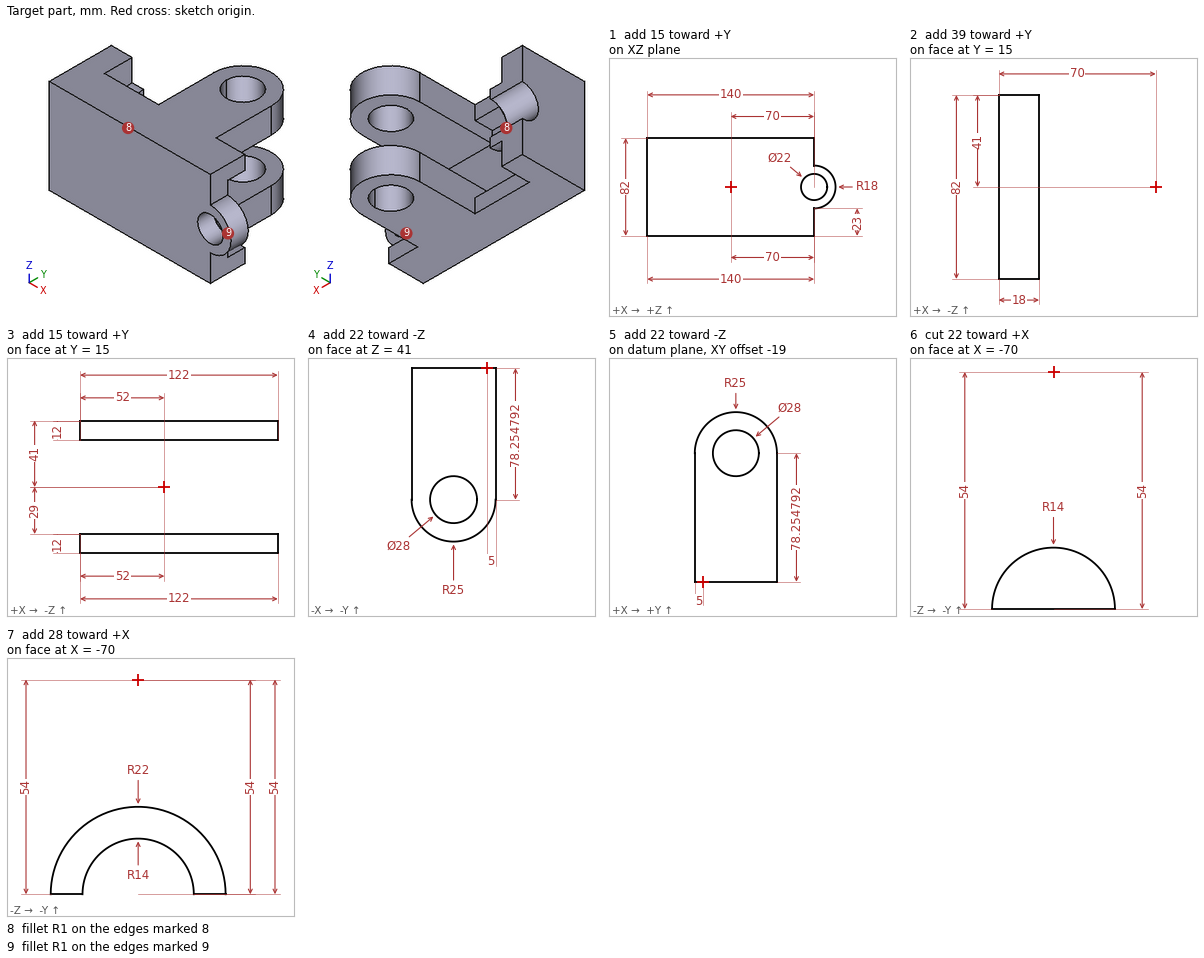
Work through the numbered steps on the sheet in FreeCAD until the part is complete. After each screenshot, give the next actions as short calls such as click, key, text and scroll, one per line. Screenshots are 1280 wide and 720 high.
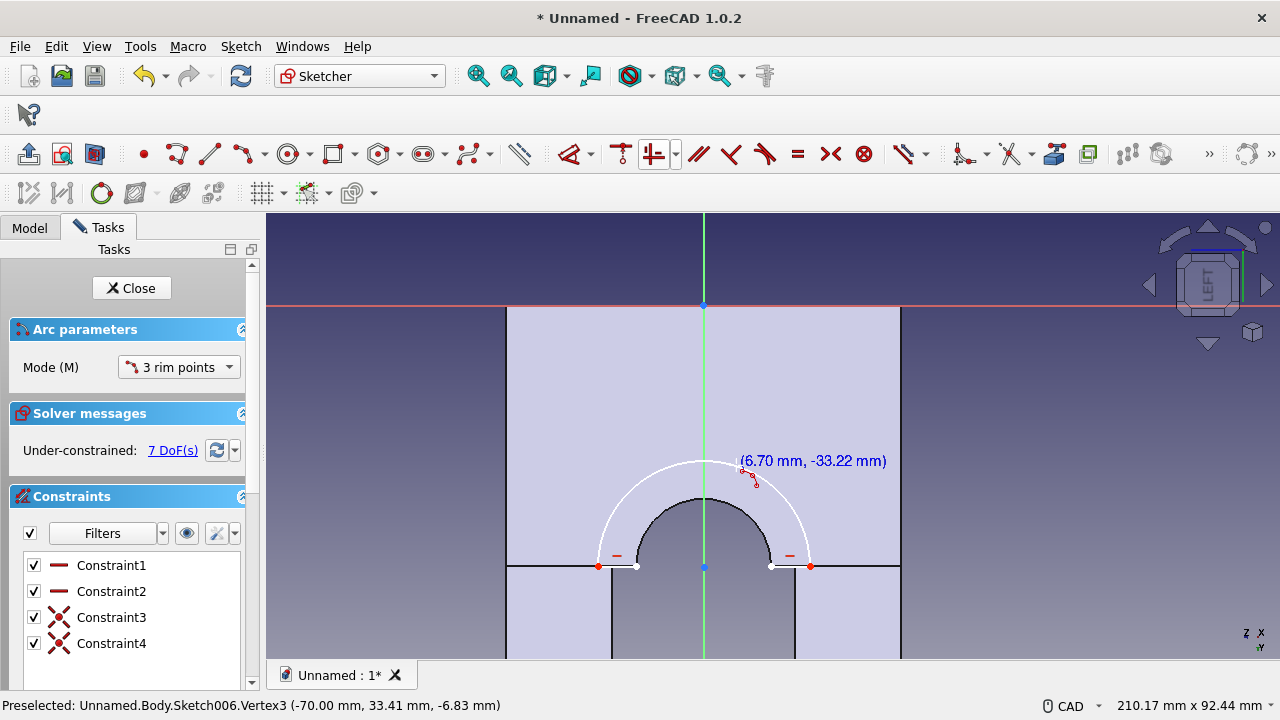
click(636, 567)
click(771, 567)
click(725, 502)
key(Escape)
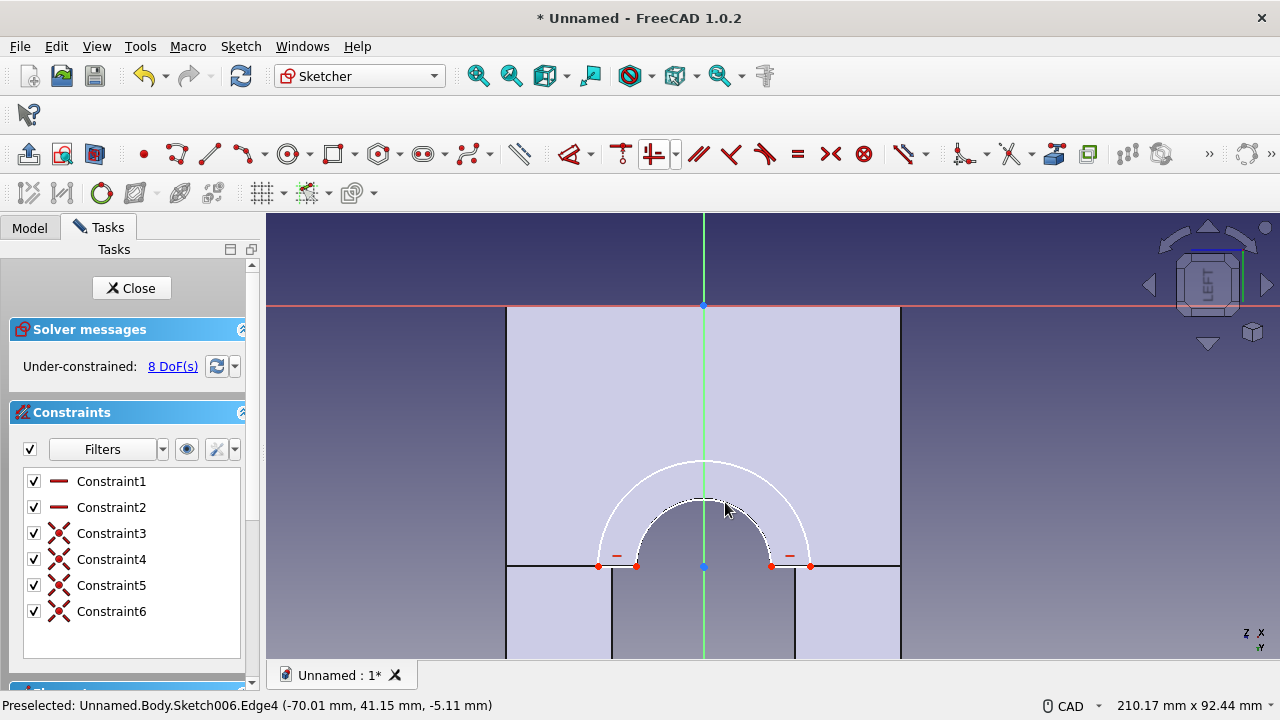
click(766, 481)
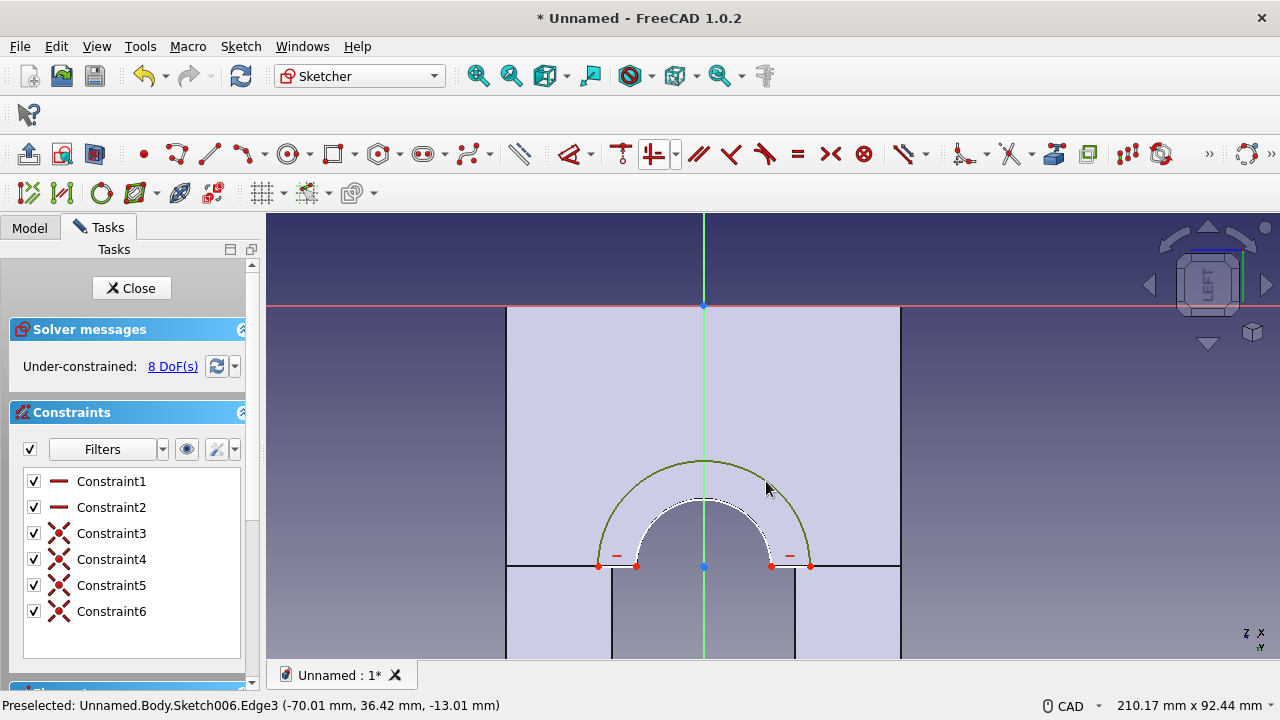
click(743, 512)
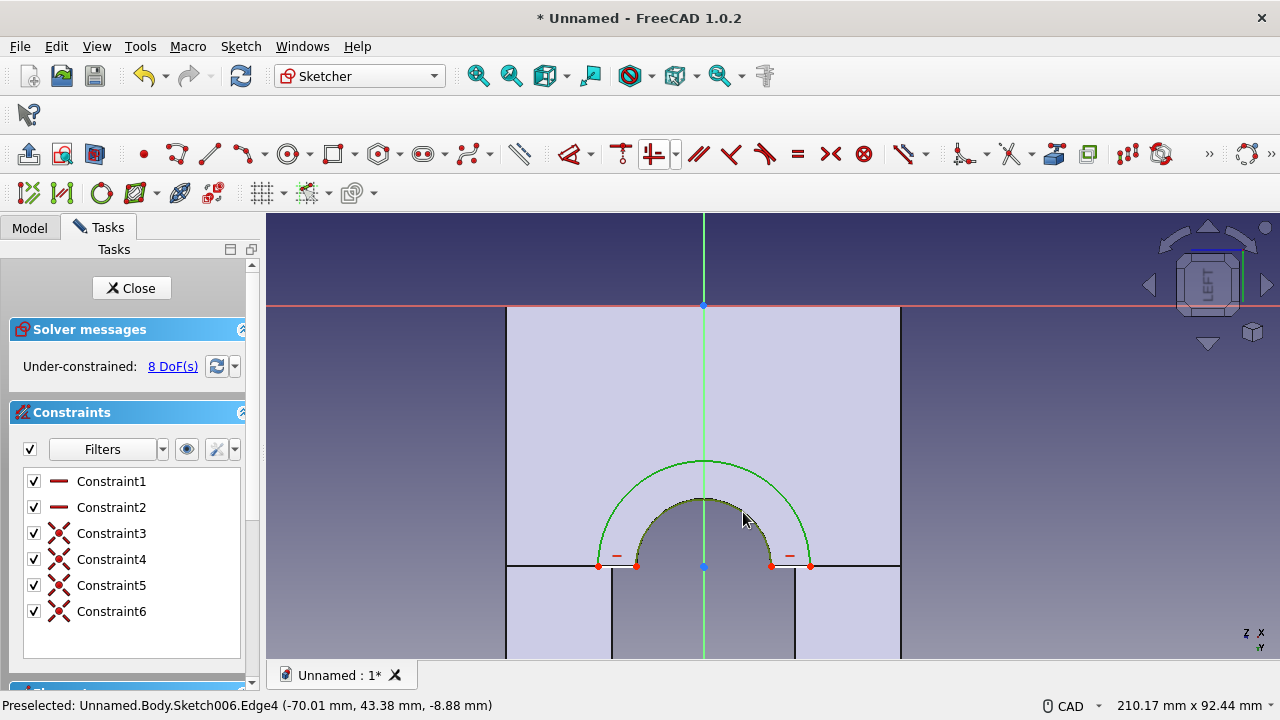
click(621, 154)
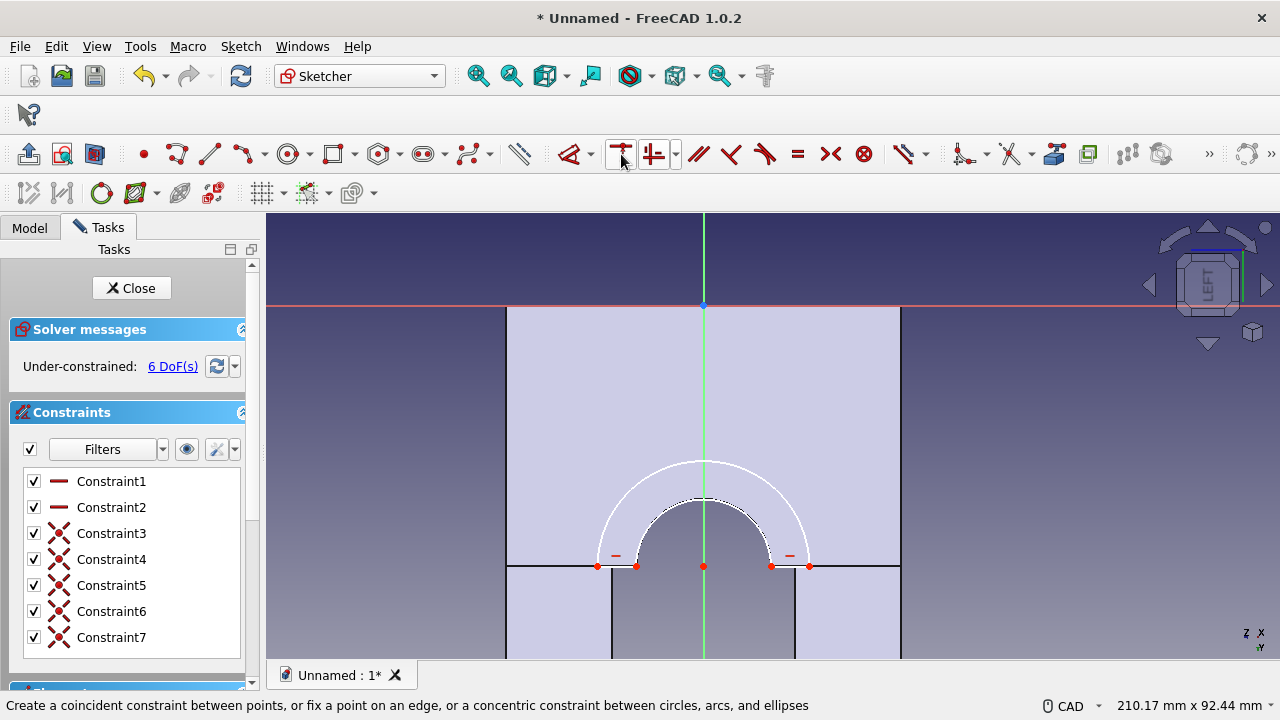
click(704, 567)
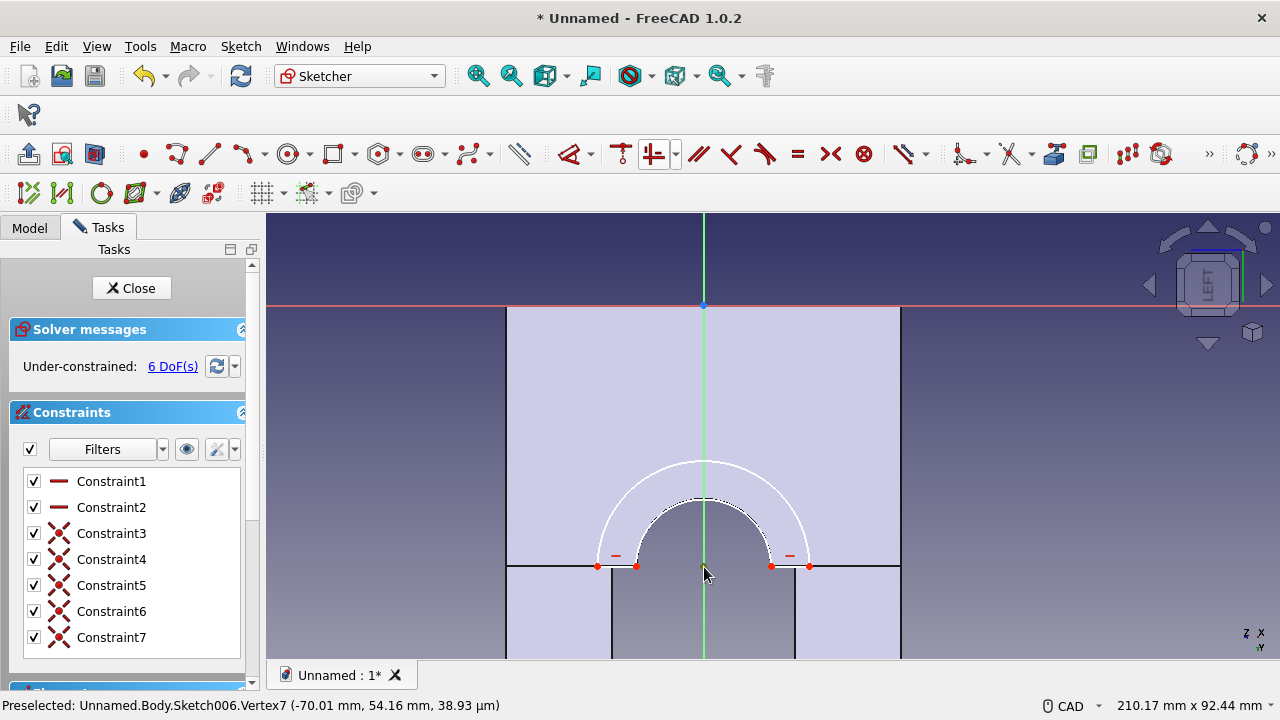
click(704, 603)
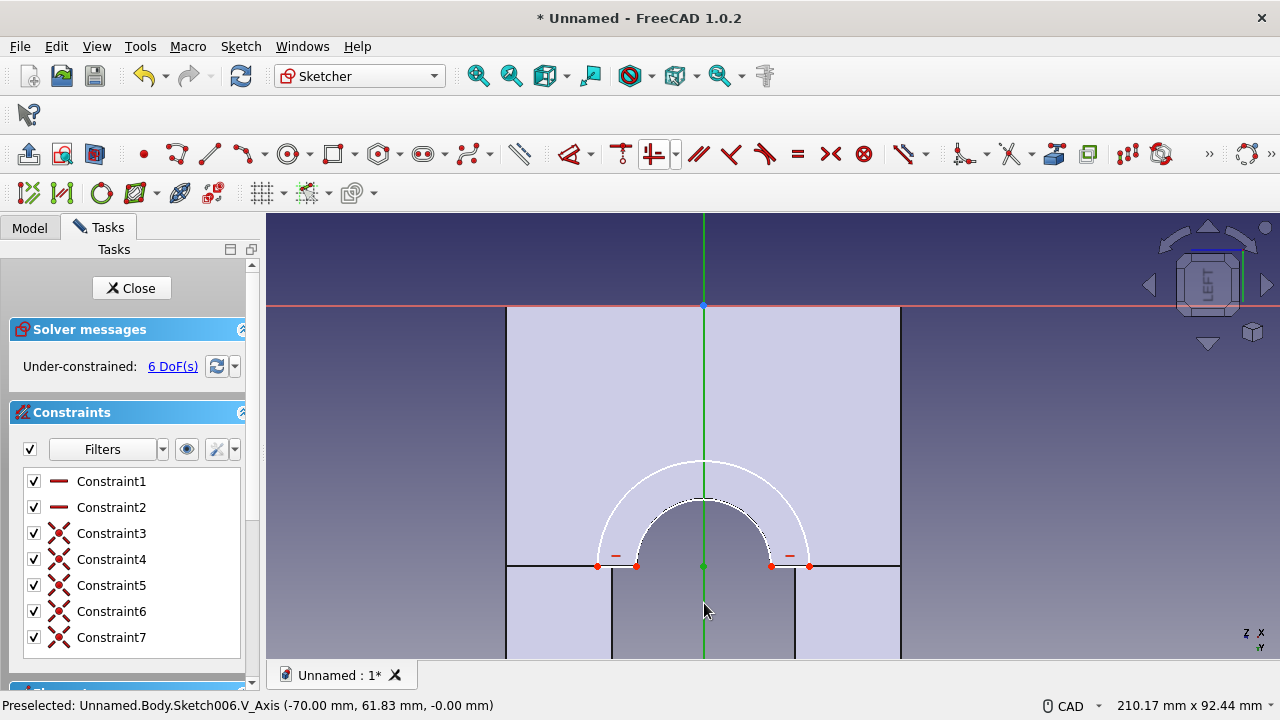
click(621, 154)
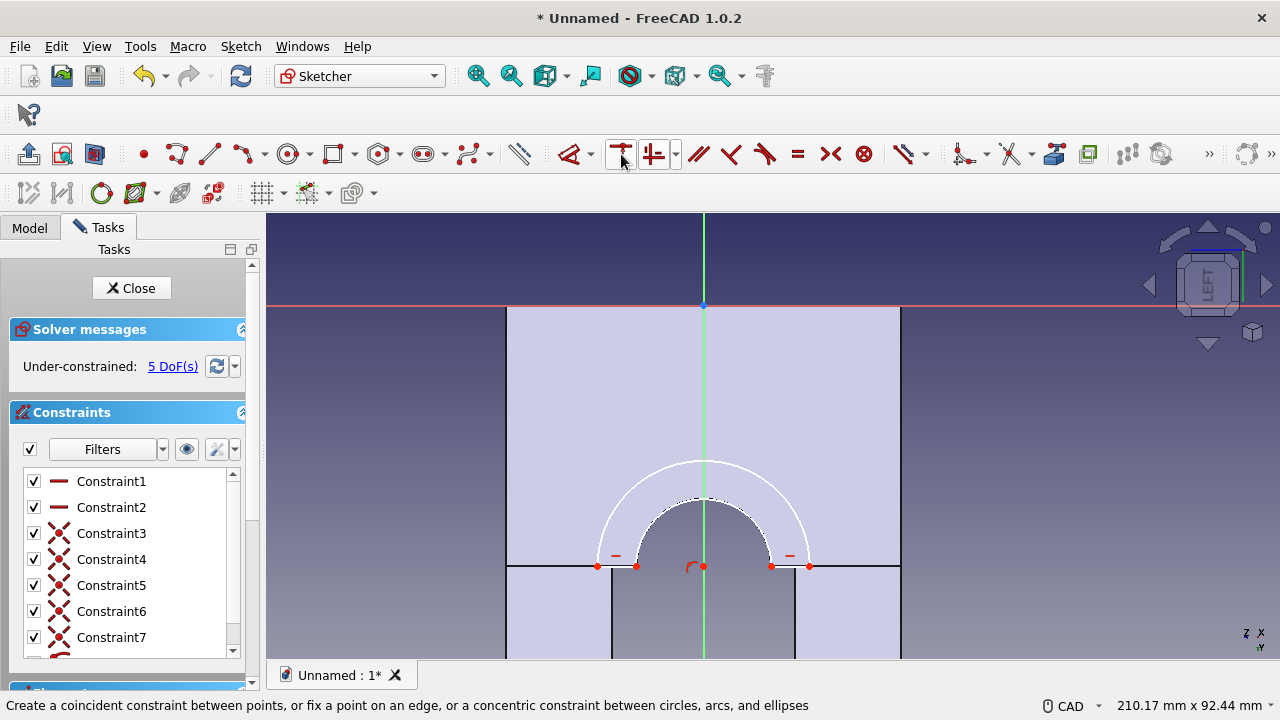
click(568, 154)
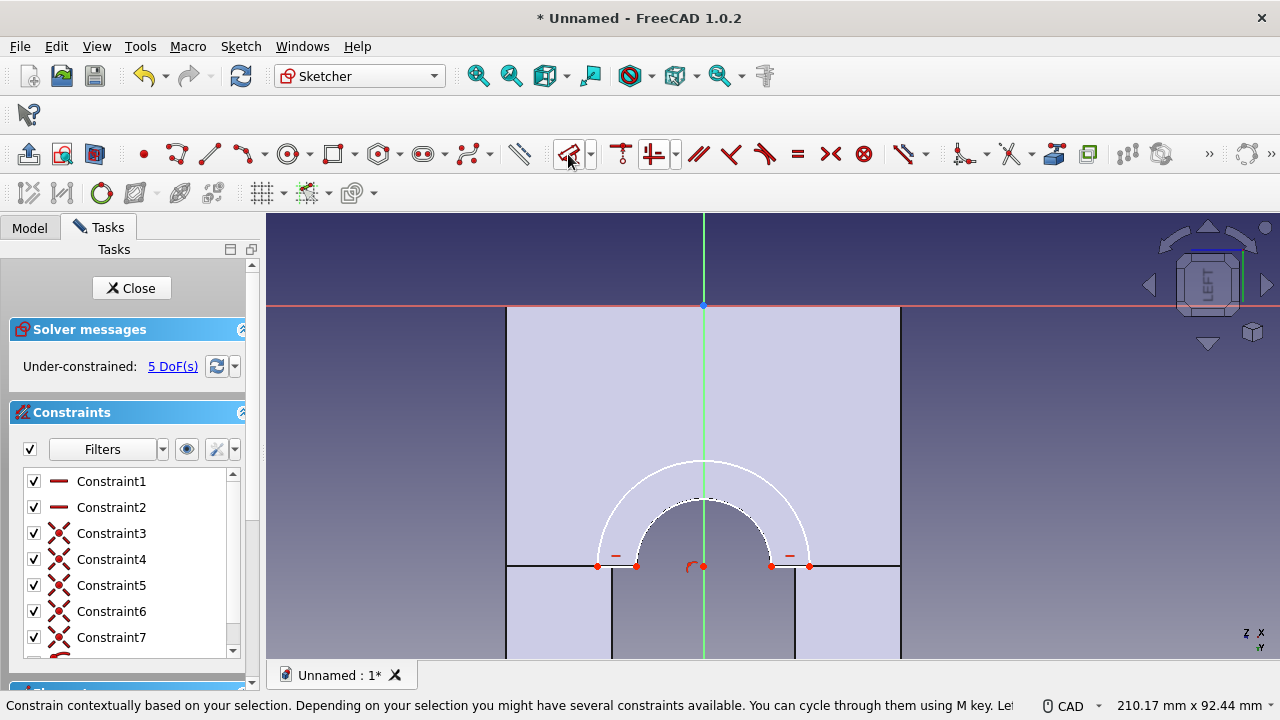
click(766, 481)
click(785, 455)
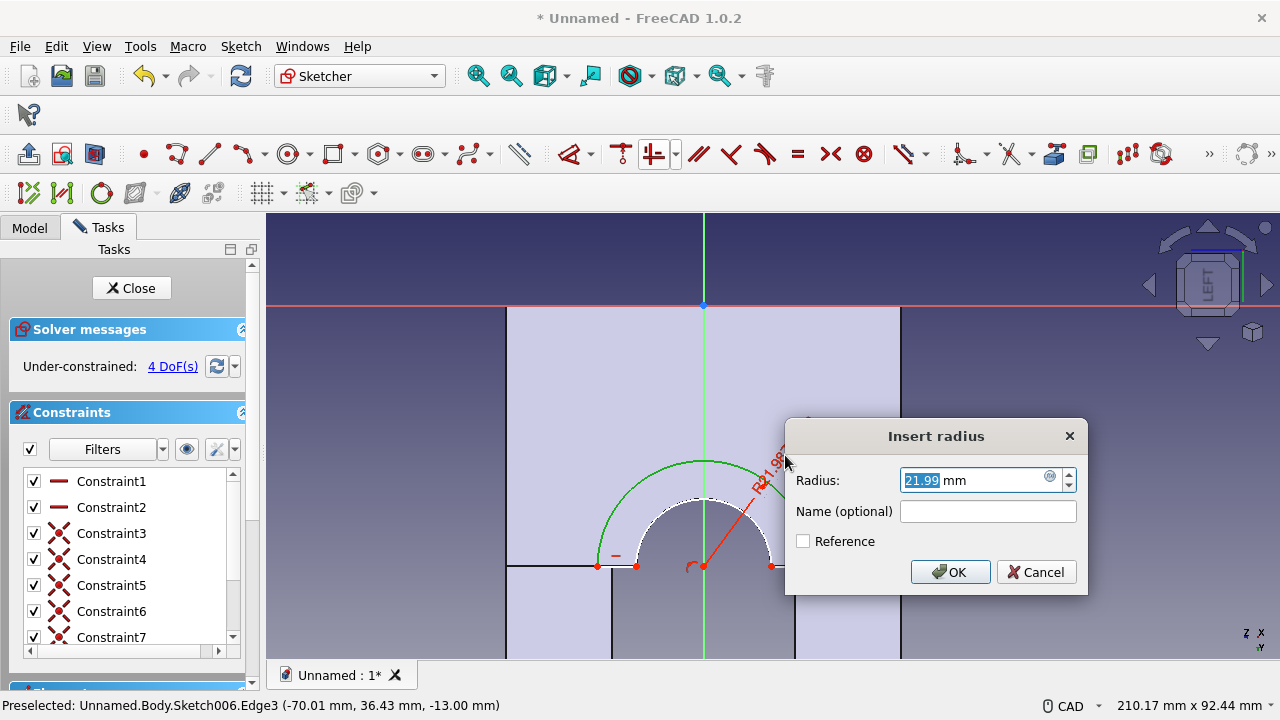
text(22)
key(Return)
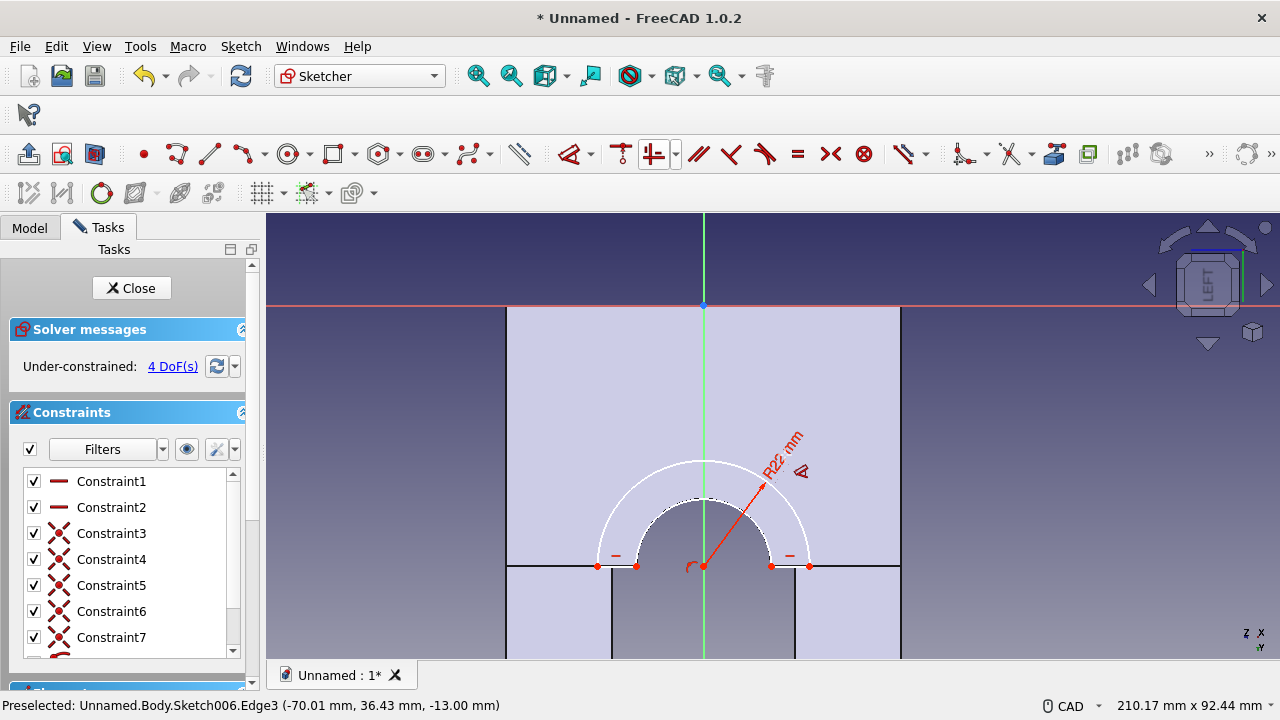
click(743, 512)
click(785, 625)